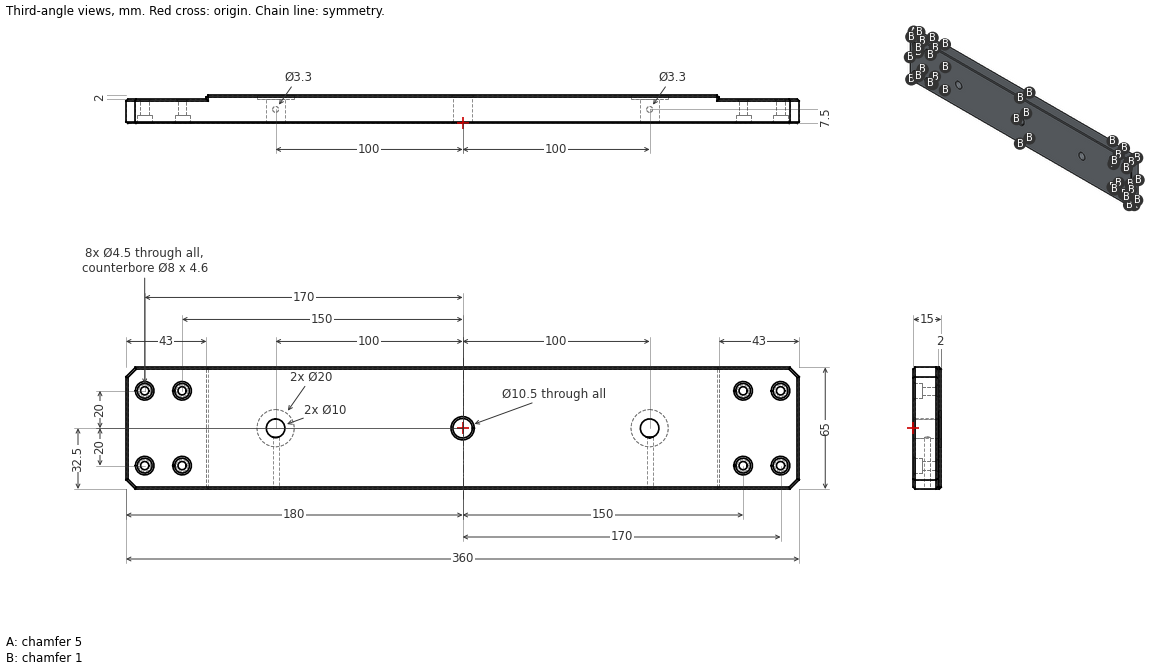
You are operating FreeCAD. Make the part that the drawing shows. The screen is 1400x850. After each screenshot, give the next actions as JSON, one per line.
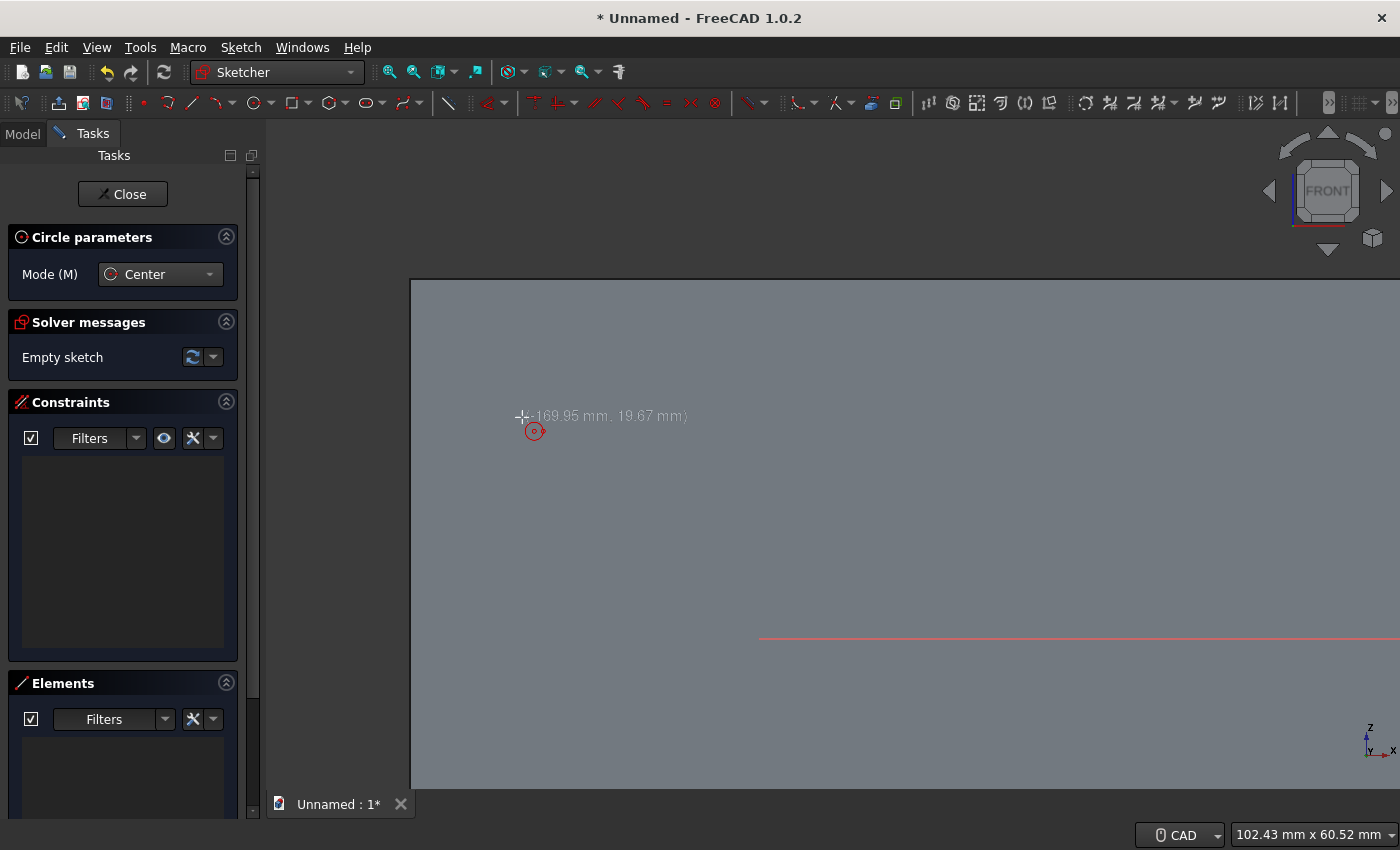
{"action": "scroll", "coordinate": [440, 417], "scroll_direction": "down", "scroll_amount": 9}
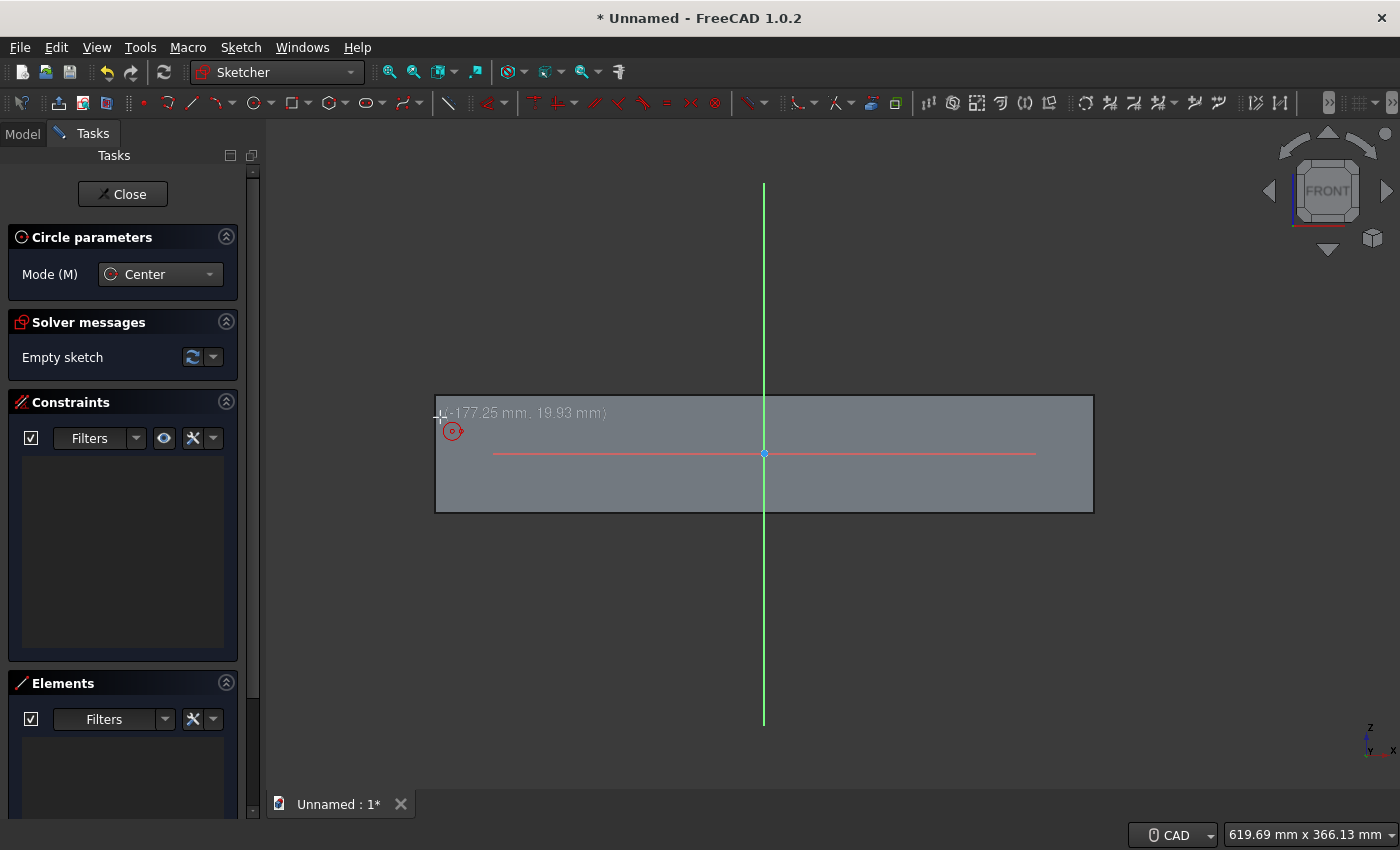
{"action": "left_click", "coordinate": [453, 417]}
{"action": "mouse_move", "coordinate": [456, 414]}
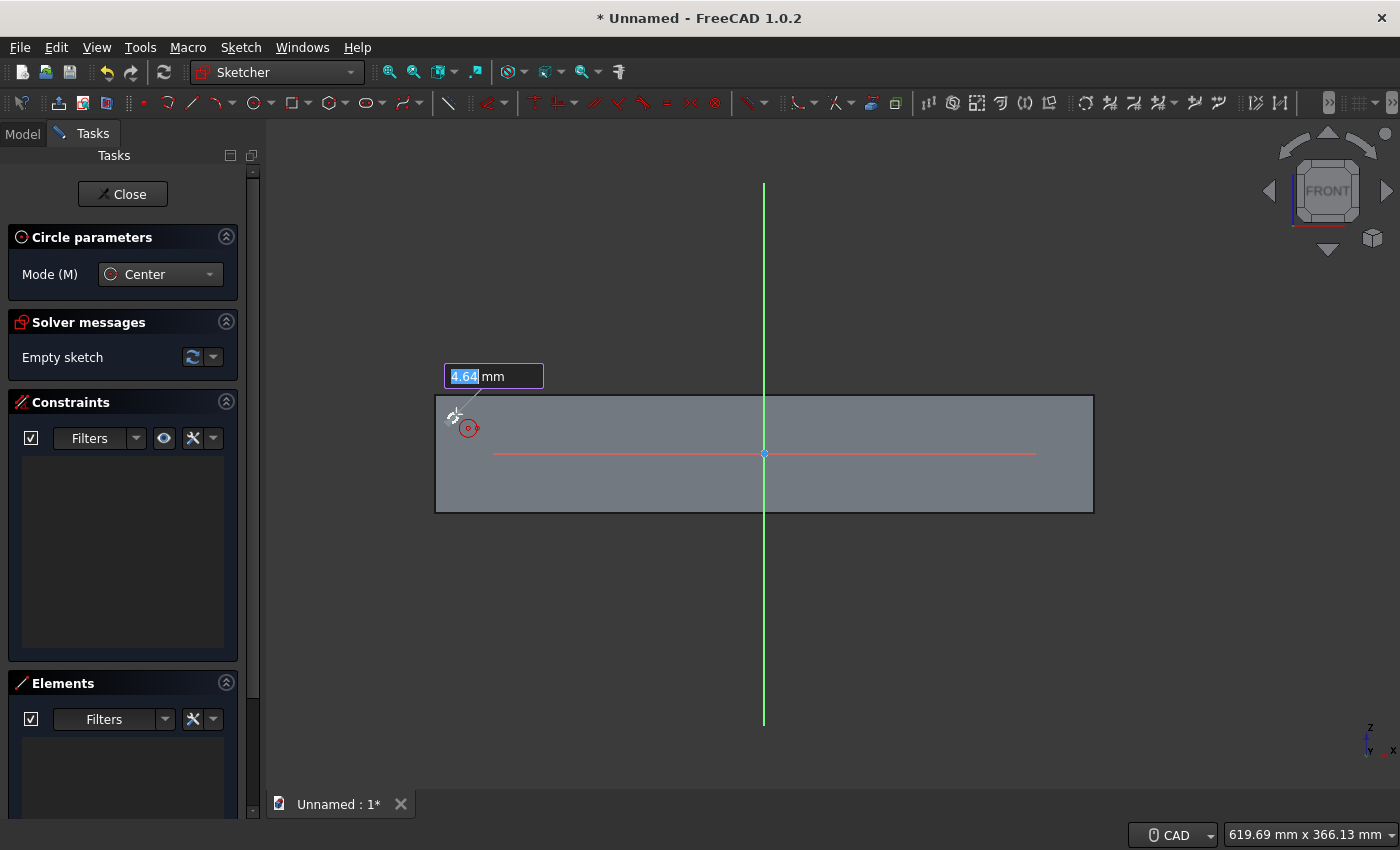
{"action": "type", "text": "4.5"}
{"action": "key", "text": "Return"}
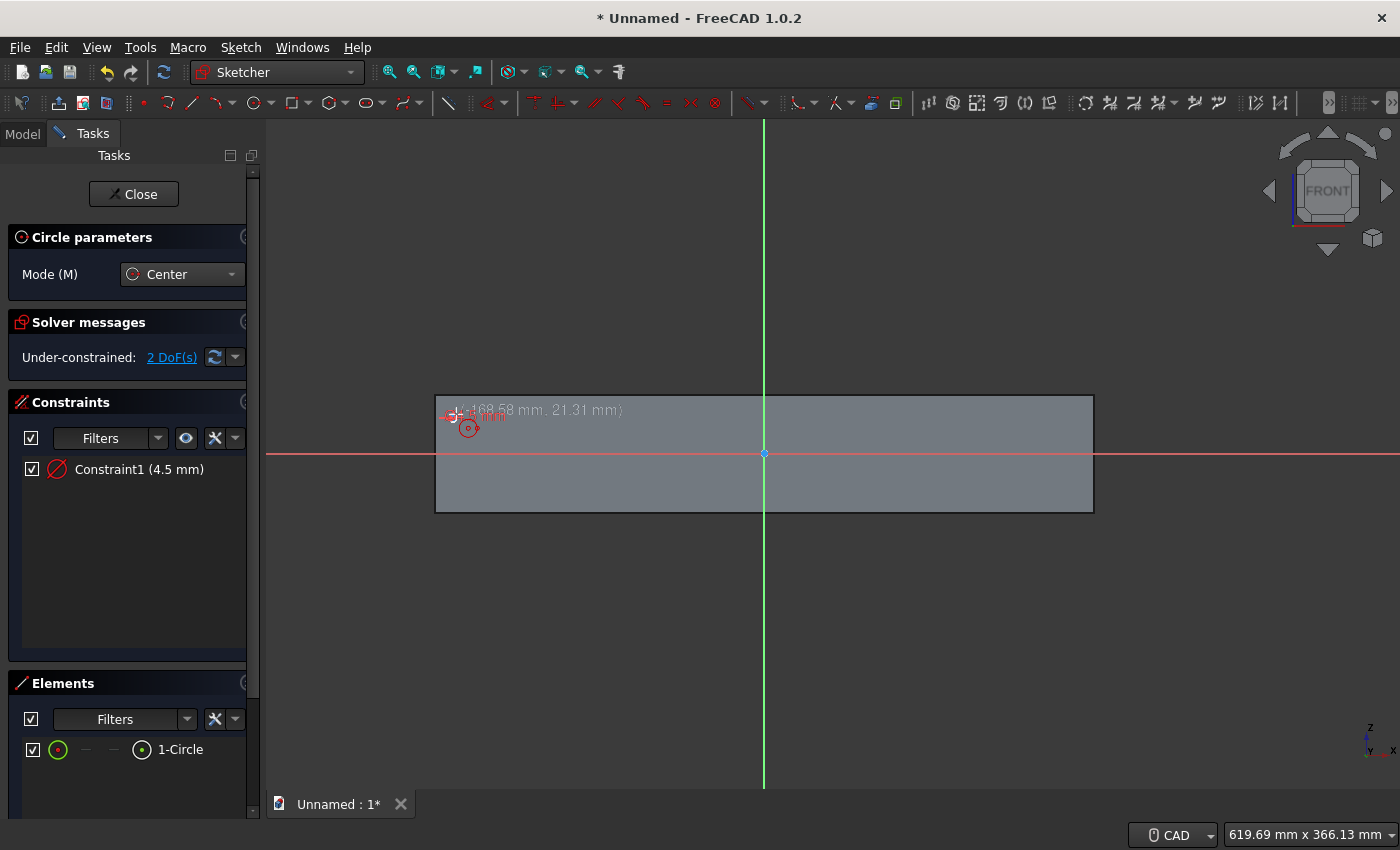
{"action": "scroll", "coordinate": [490, 417], "scroll_direction": "up", "scroll_amount": 9}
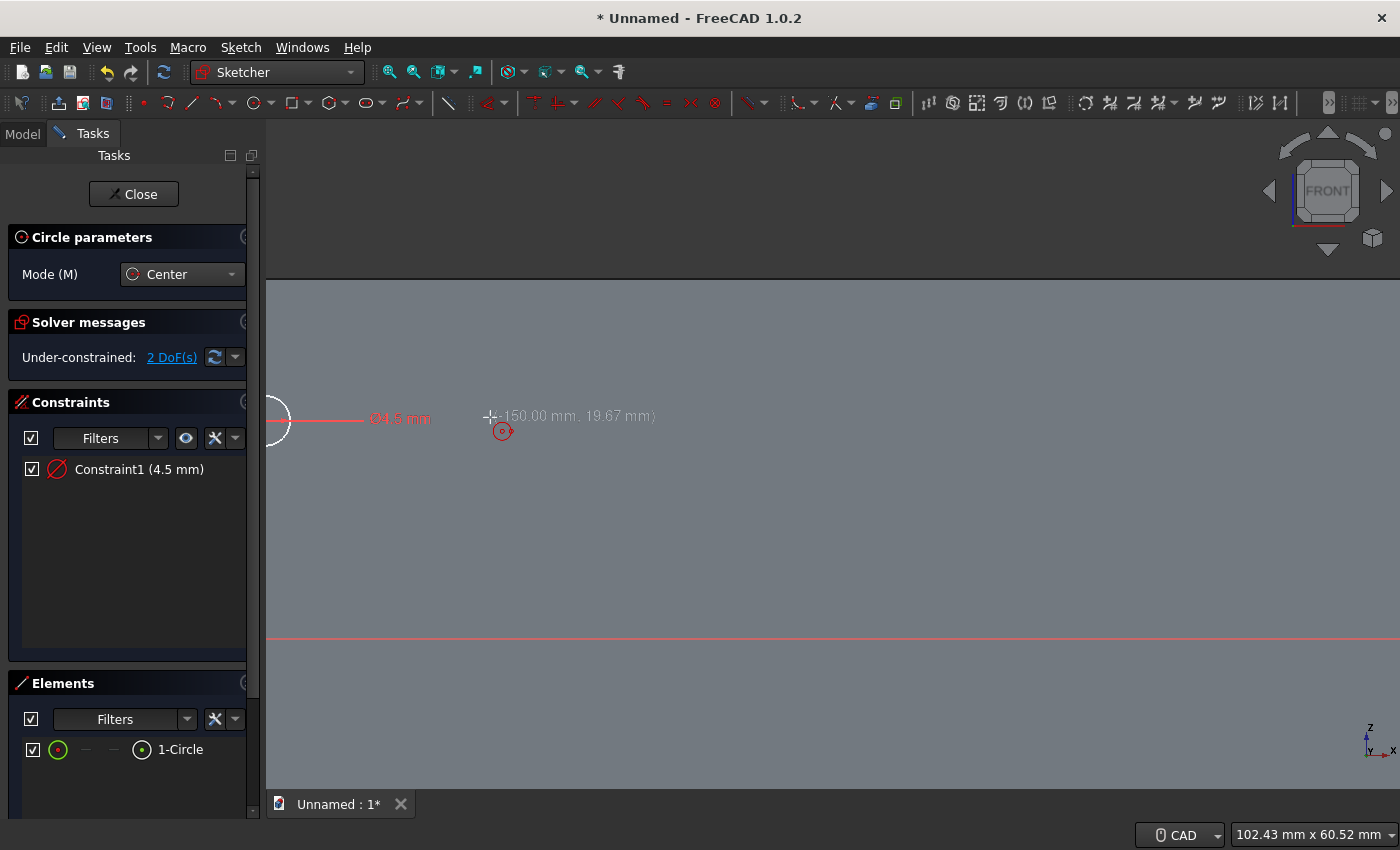
{"action": "scroll", "coordinate": [490, 417], "scroll_direction": "down", "scroll_amount": 9}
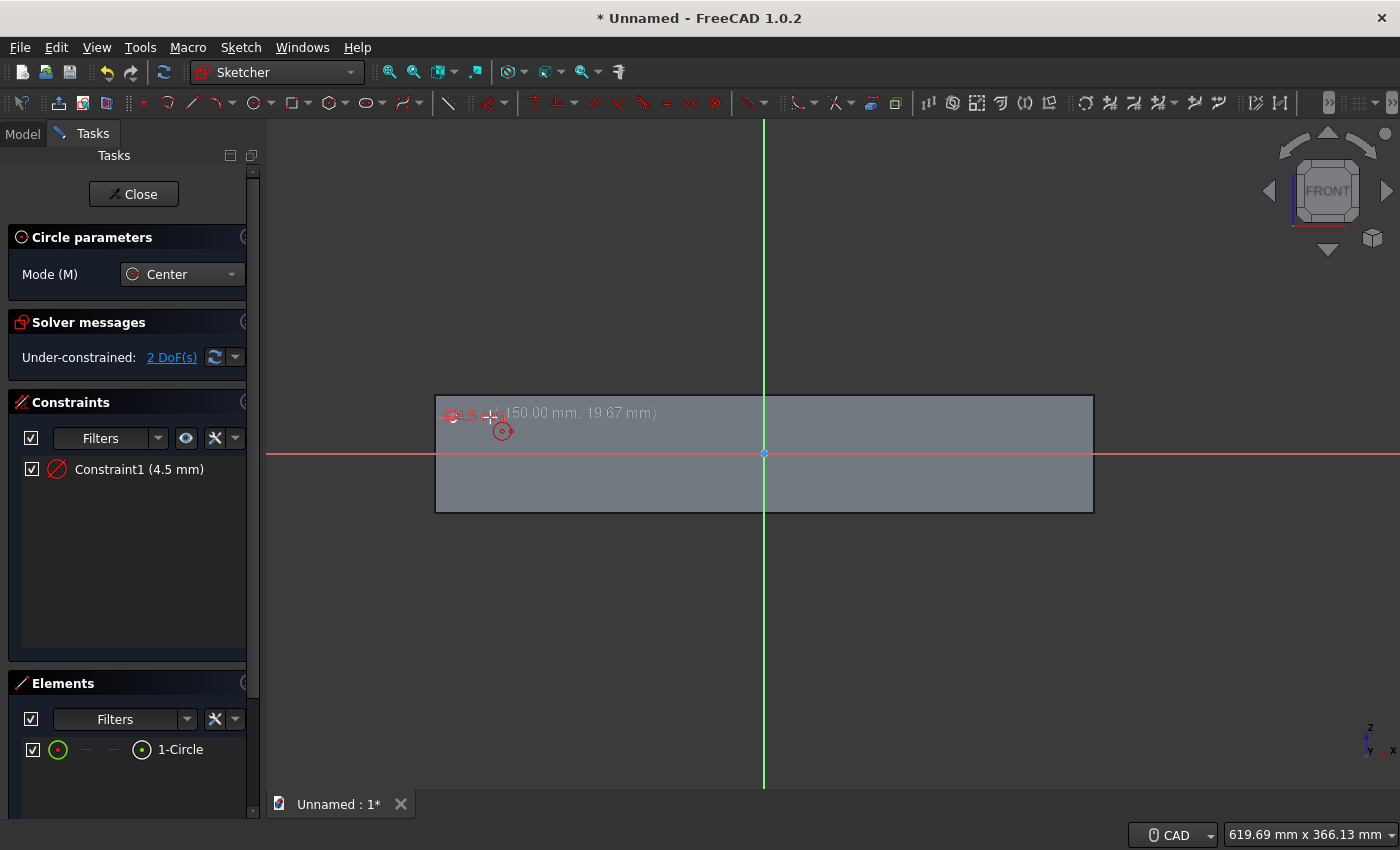
{"action": "left_click", "coordinate": [490, 417]}
{"action": "mouse_move", "coordinate": [493, 414]}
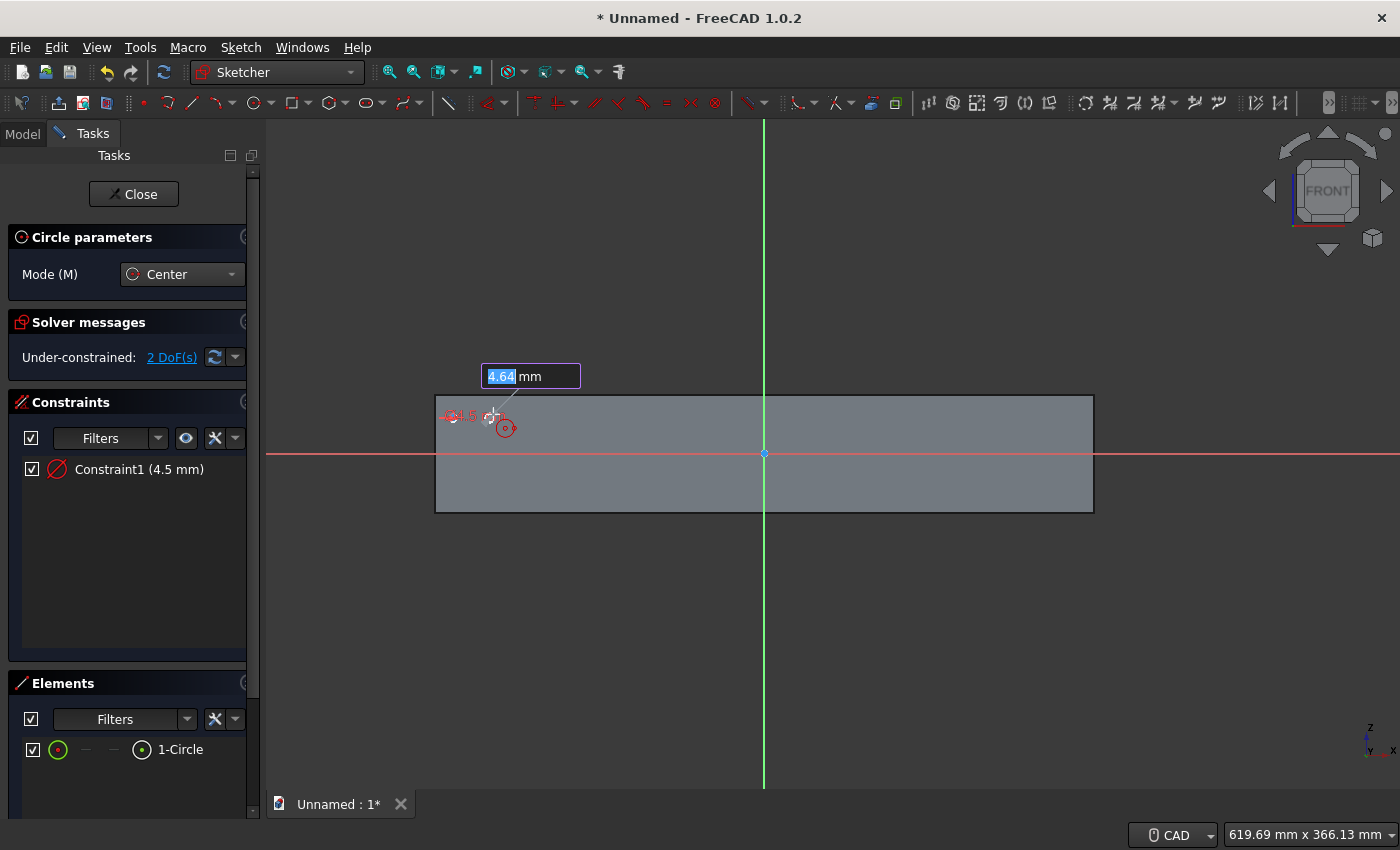
{"action": "type", "text": "4.5"}
{"action": "key", "text": "Return"}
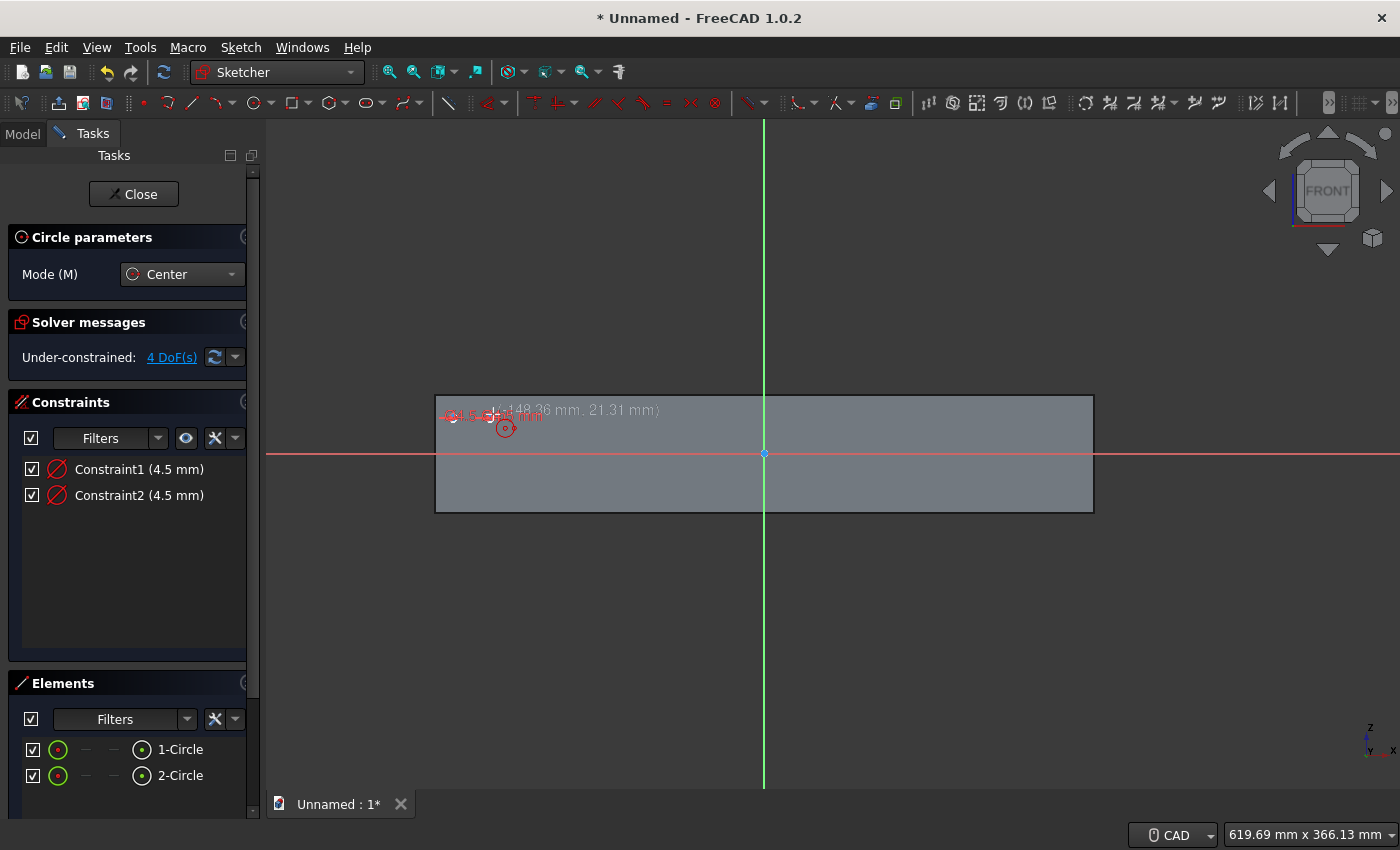
{"action": "scroll", "coordinate": [453, 491], "scroll_direction": "up", "scroll_amount": 9}